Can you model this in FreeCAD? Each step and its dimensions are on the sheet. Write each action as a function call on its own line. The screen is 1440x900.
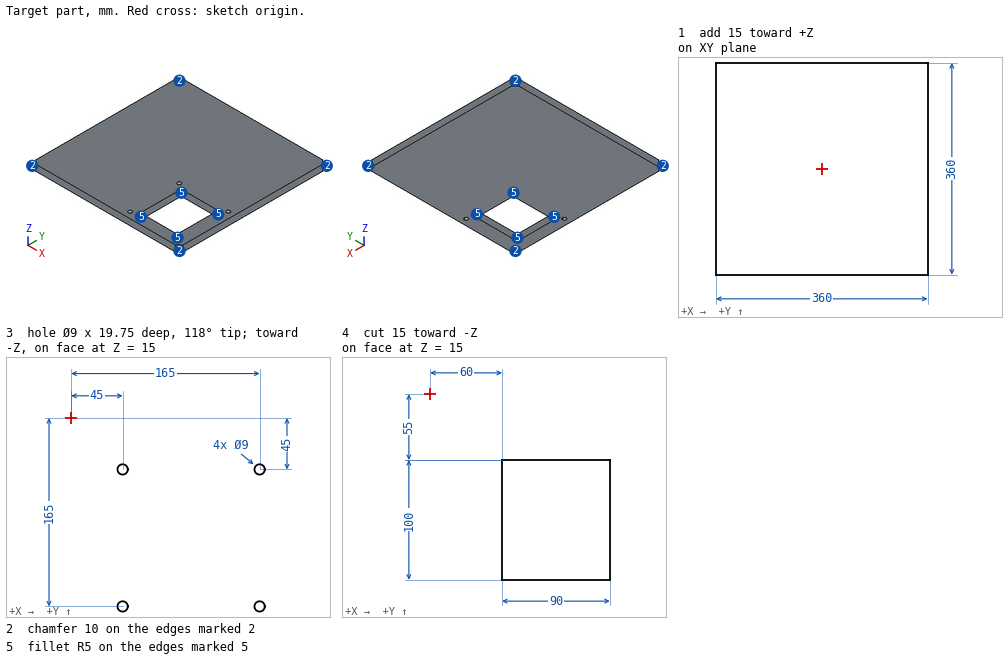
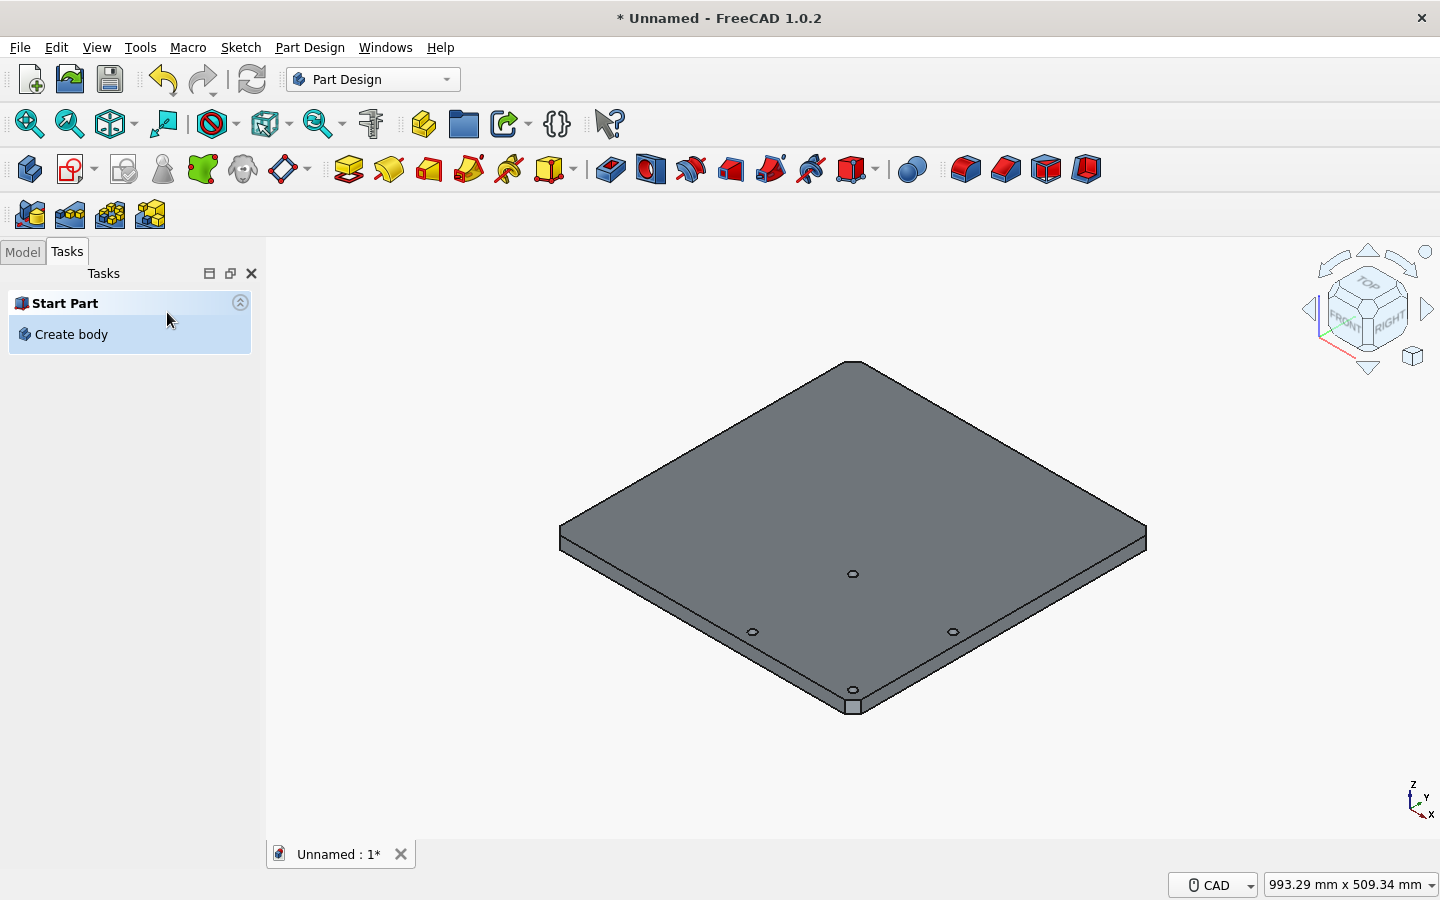
click(853, 480)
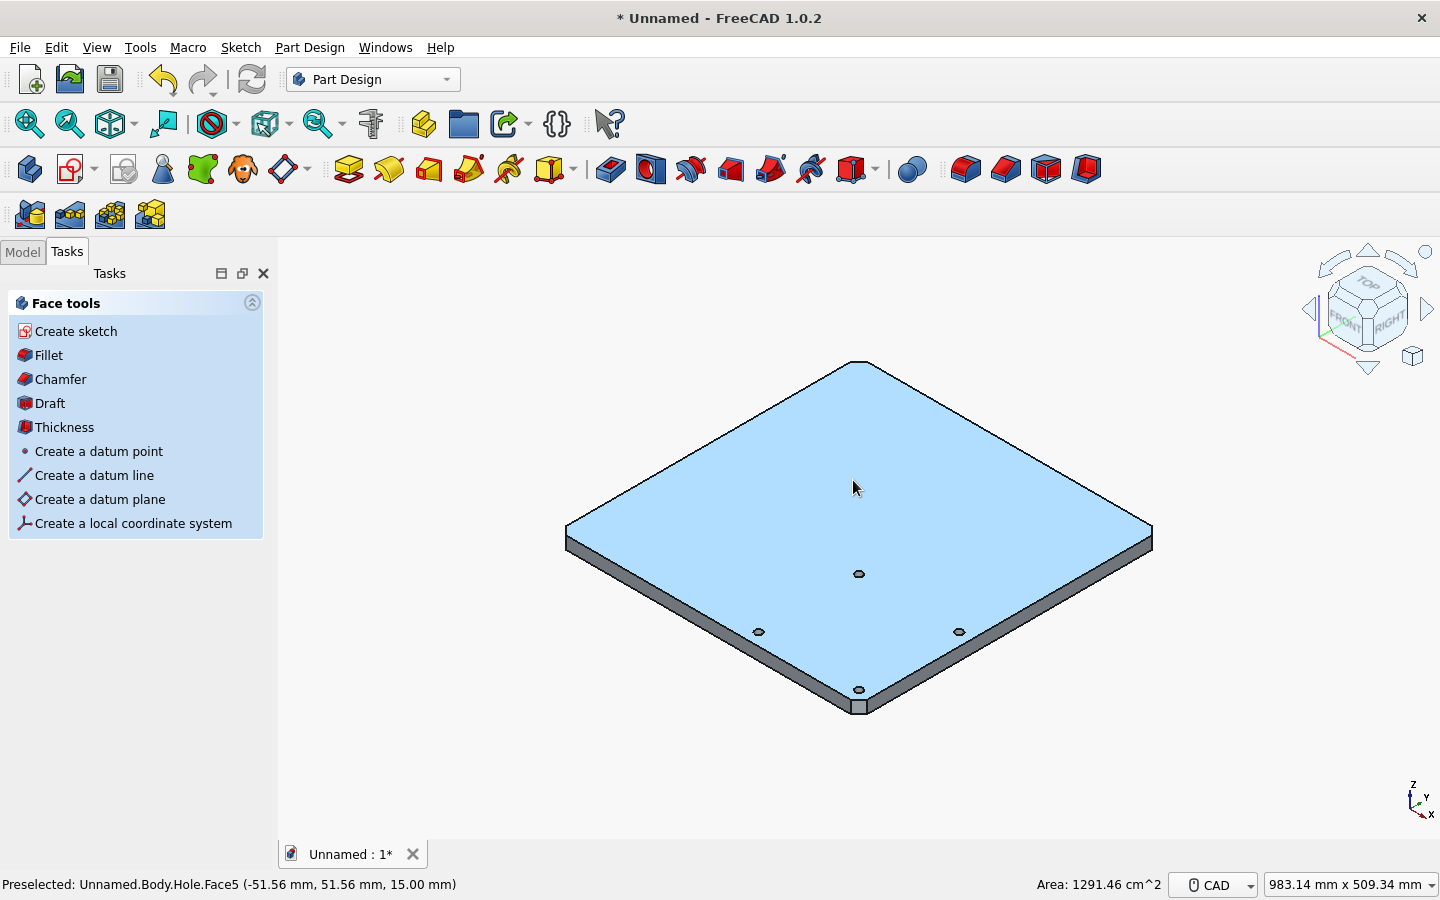
click(70, 170)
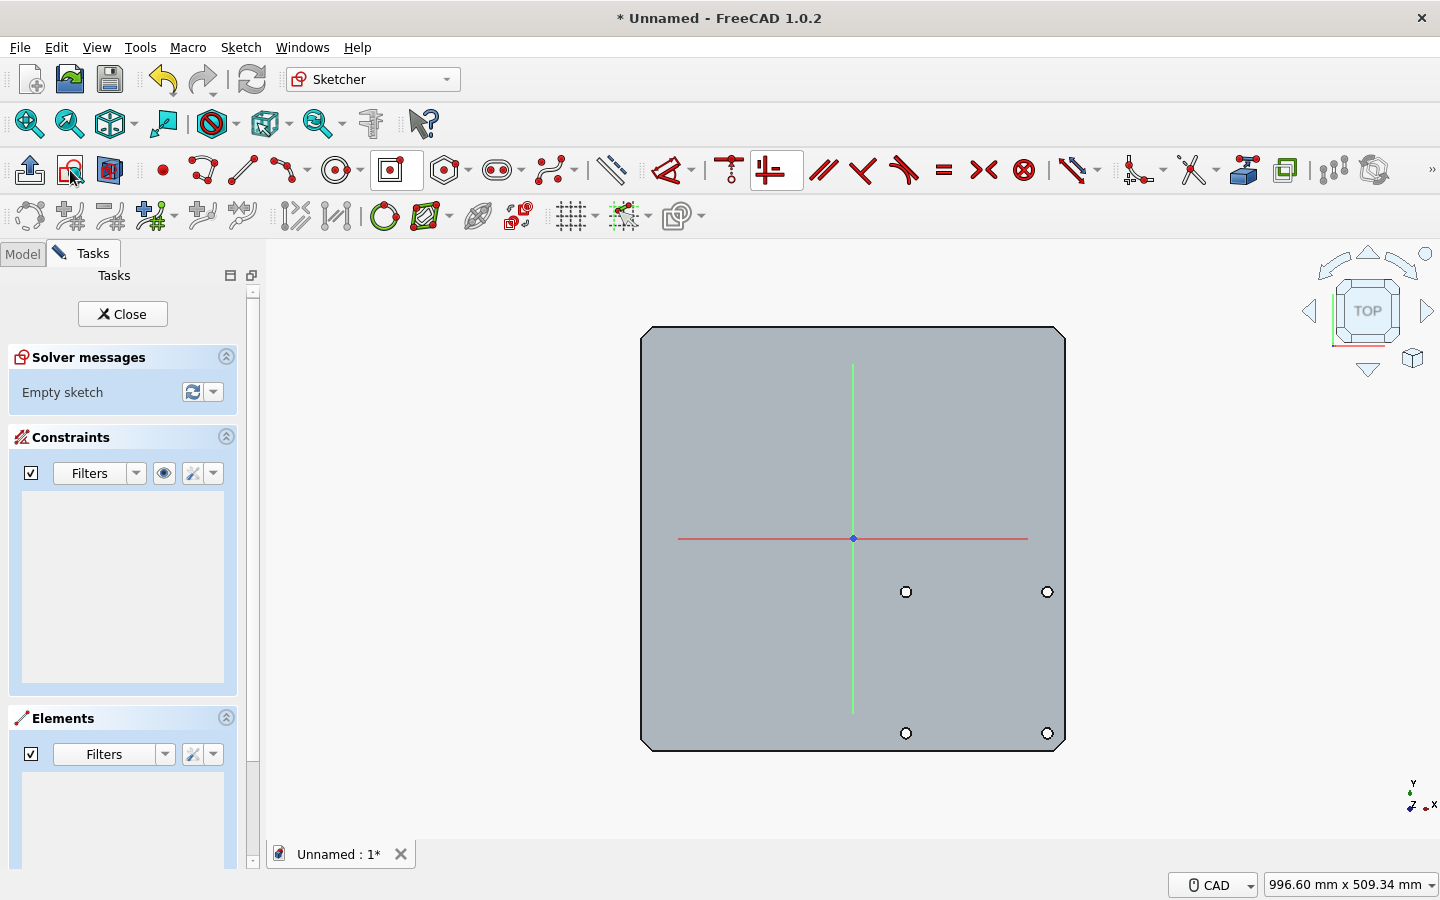
scroll(1069, 705, up, 4)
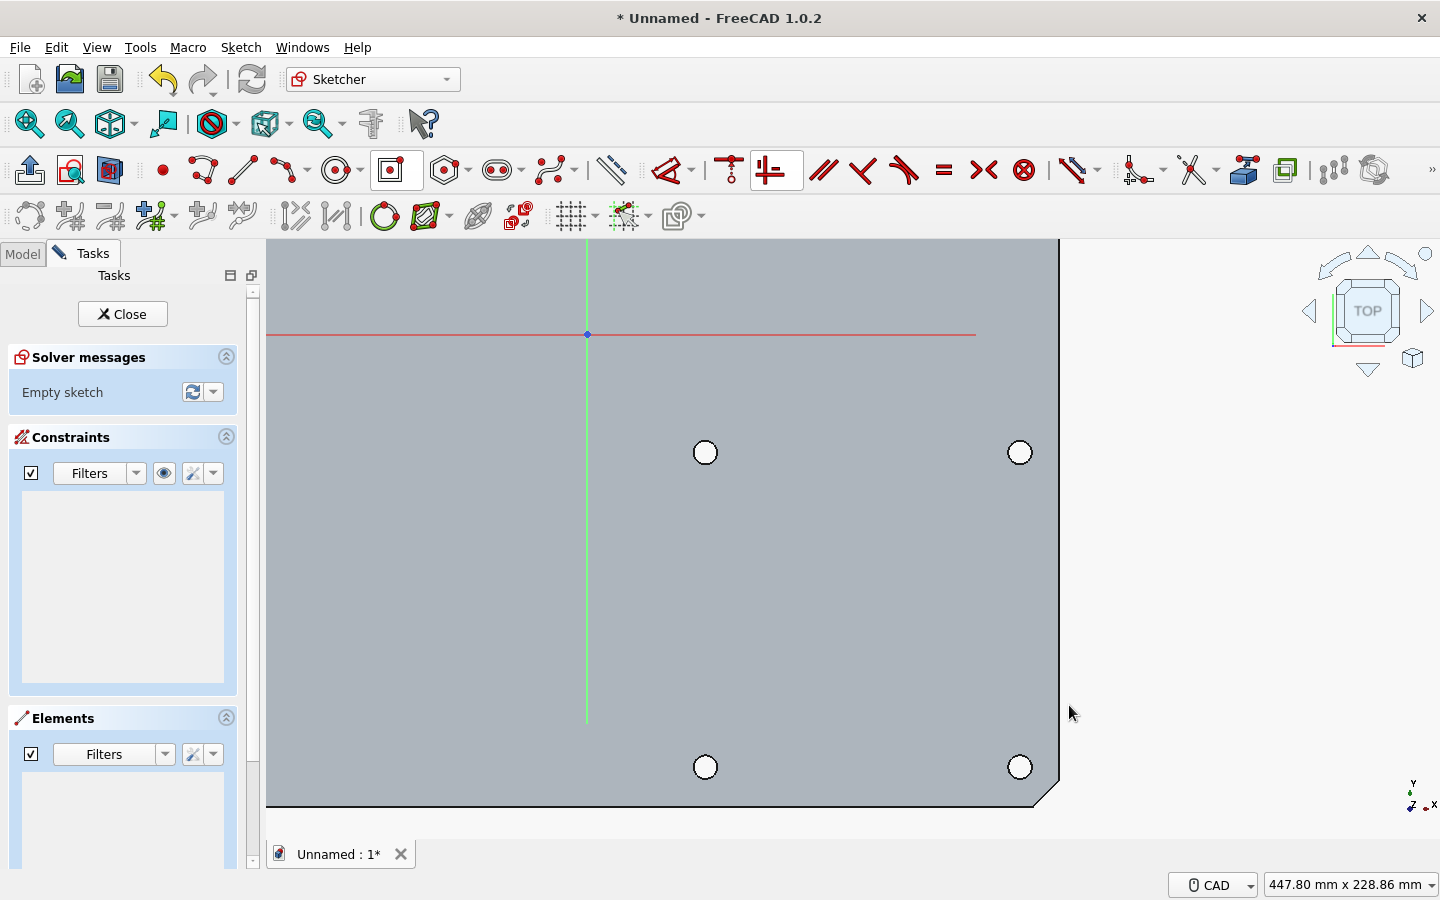
key(g)
key(r)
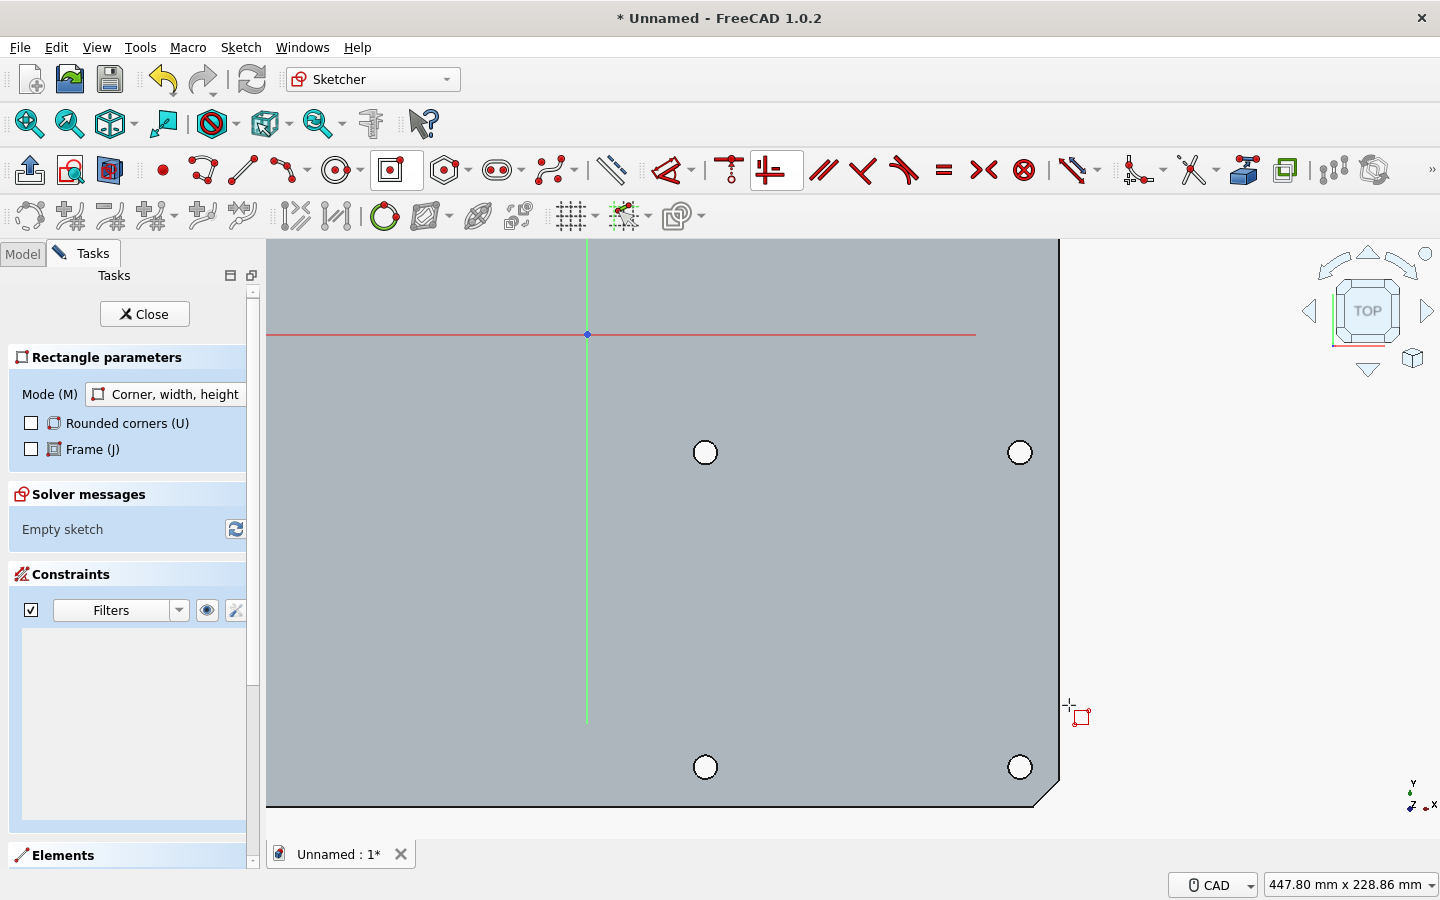
click(745, 479)
click(981, 741)
key(Escape)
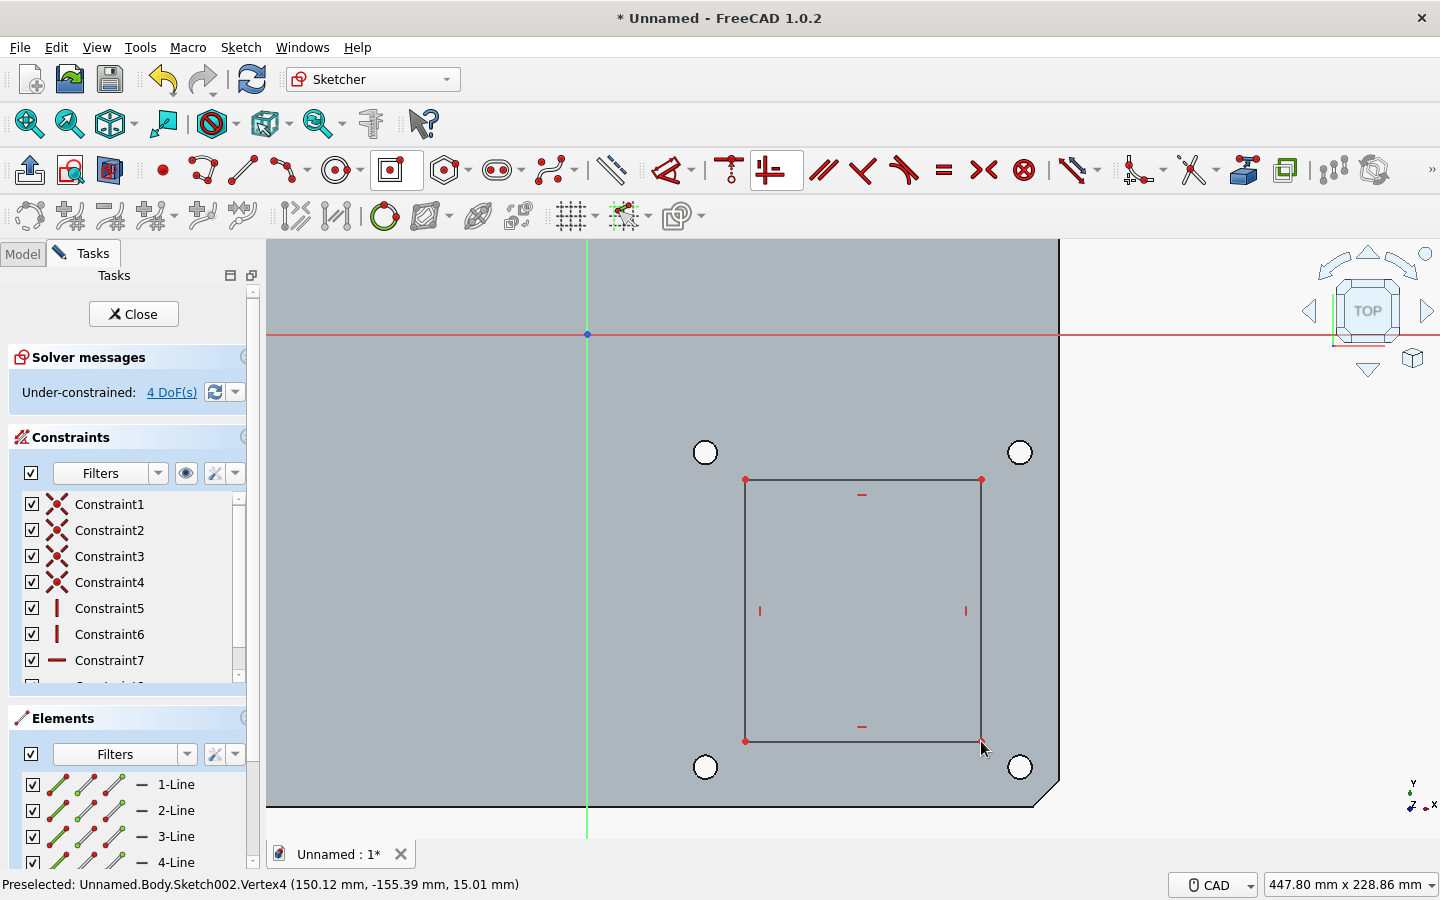
key(d)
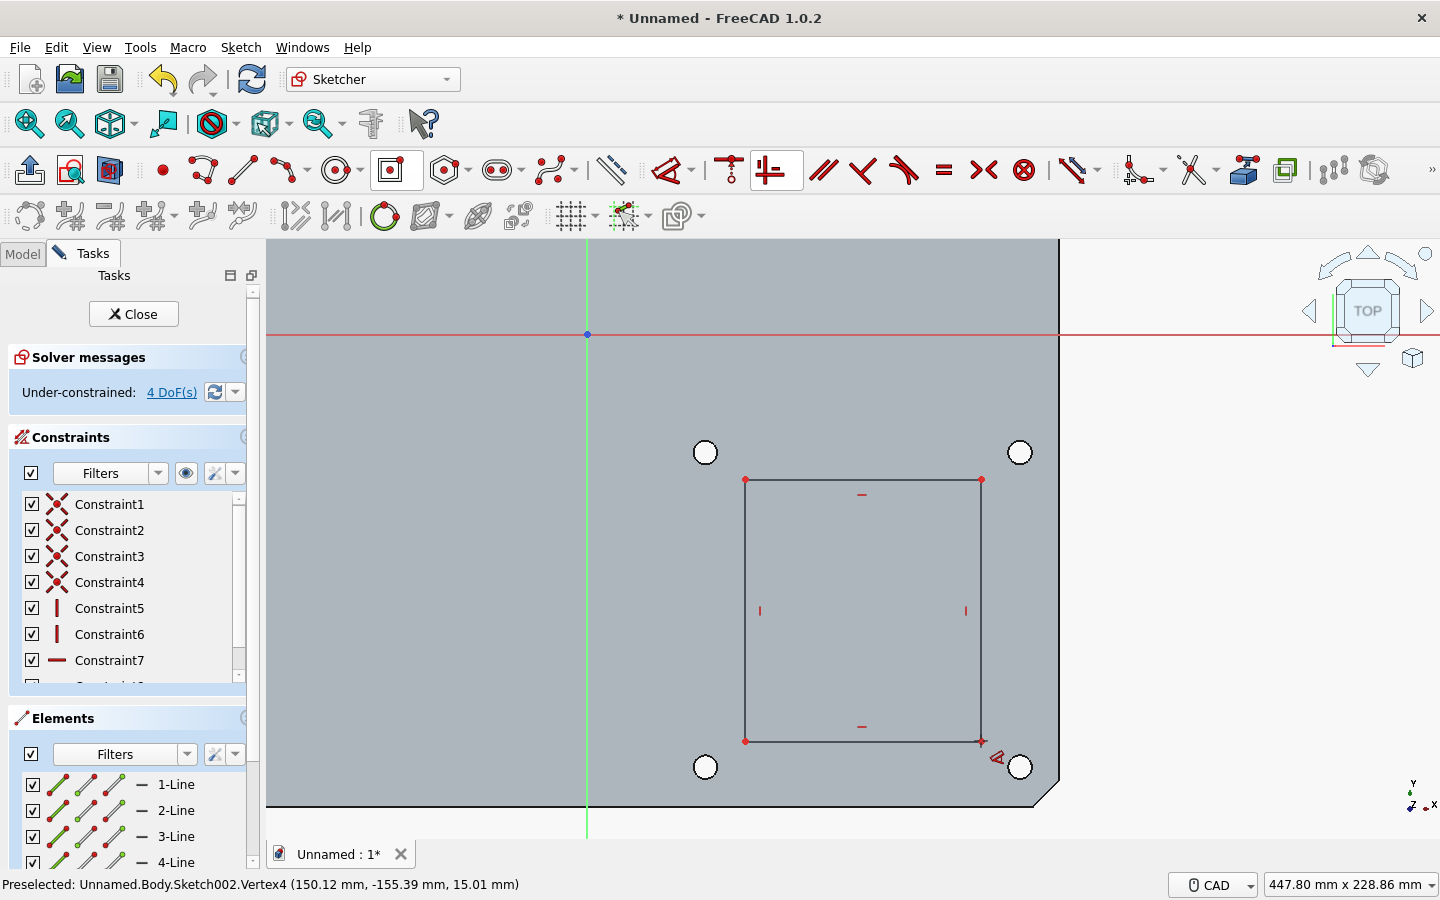
click(816, 742)
click(863, 776)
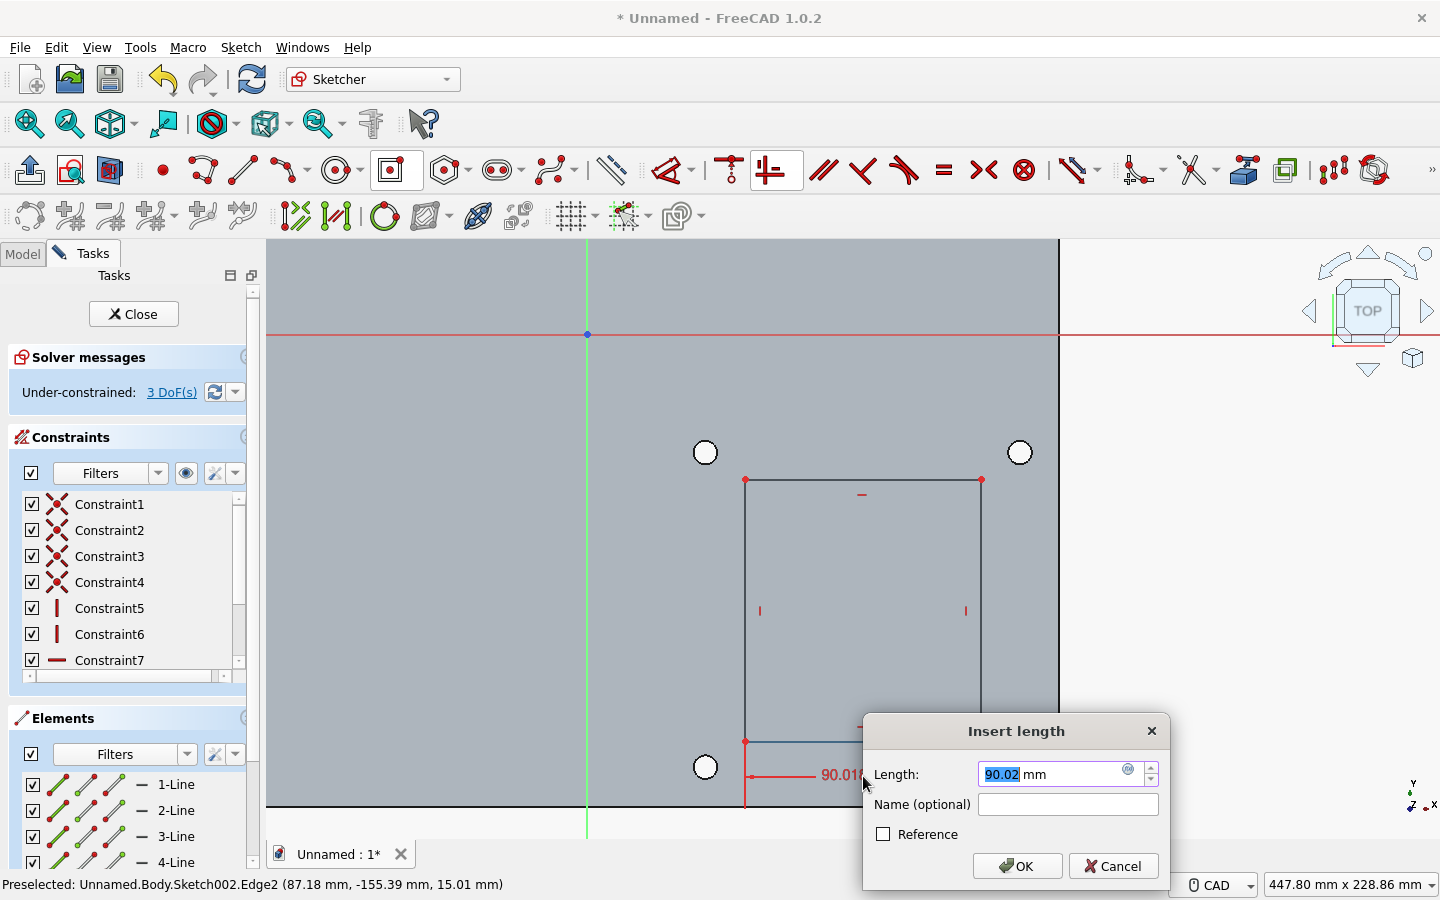
text(90)
key(Return)